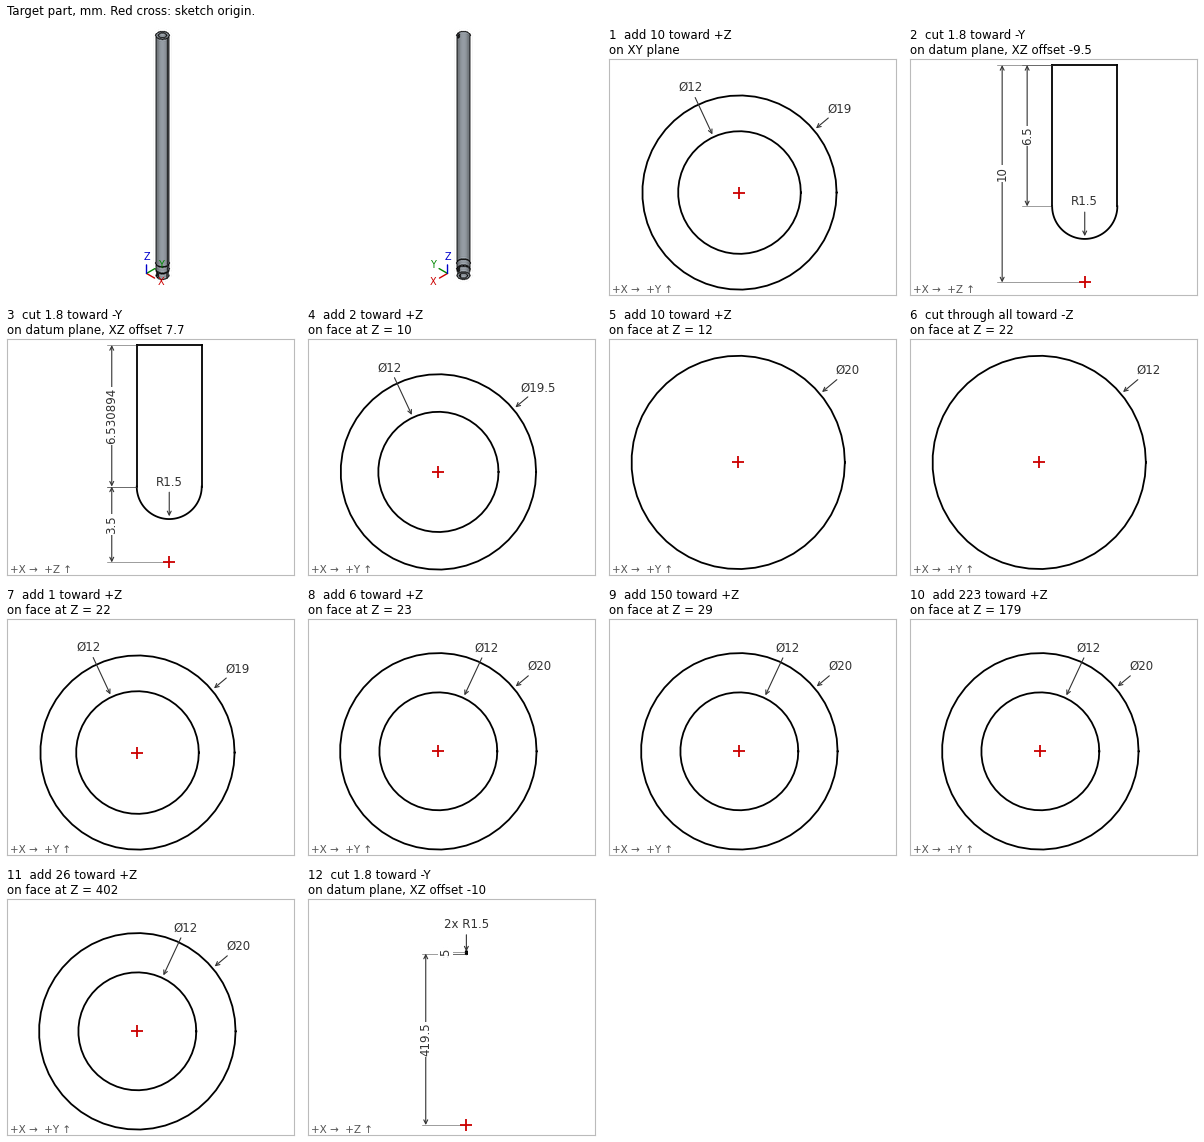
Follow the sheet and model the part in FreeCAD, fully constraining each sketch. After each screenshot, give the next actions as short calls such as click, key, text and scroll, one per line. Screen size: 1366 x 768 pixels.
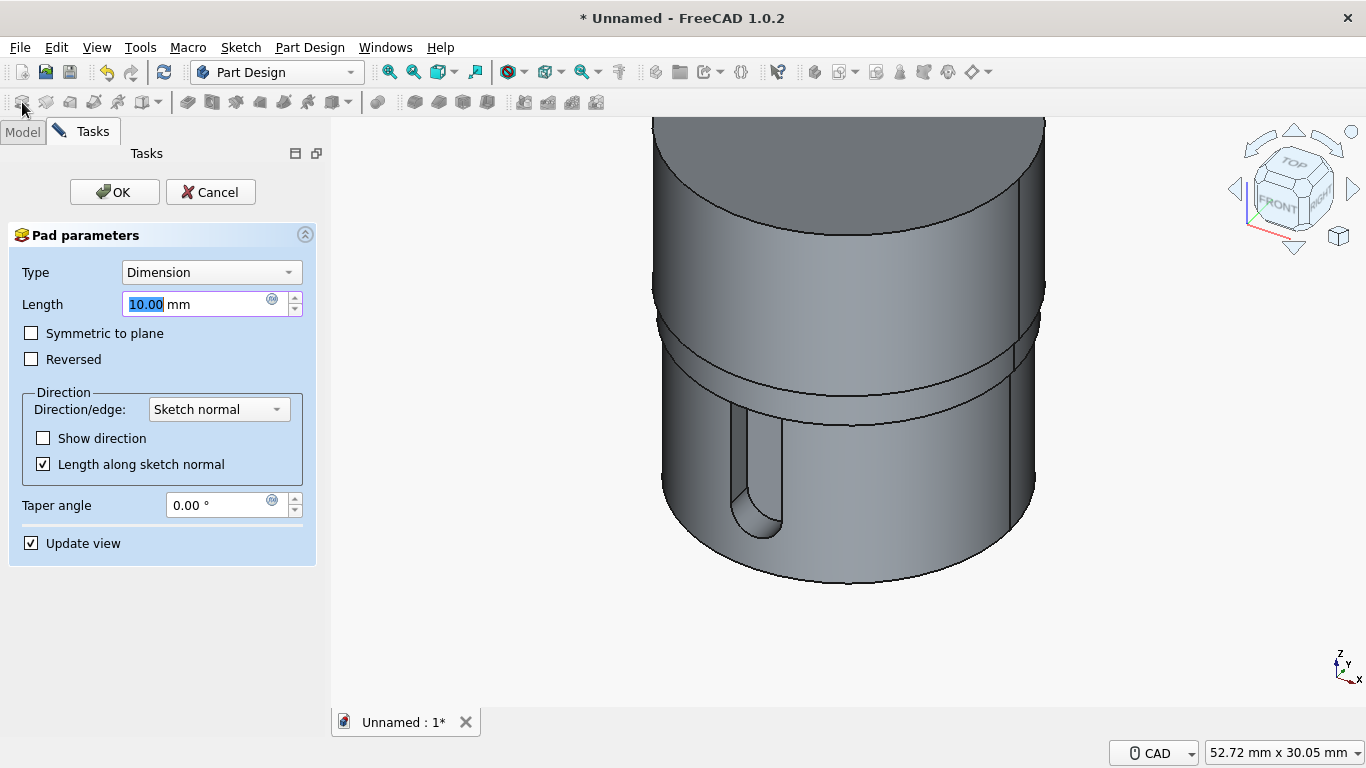
text(10)
key(Tab)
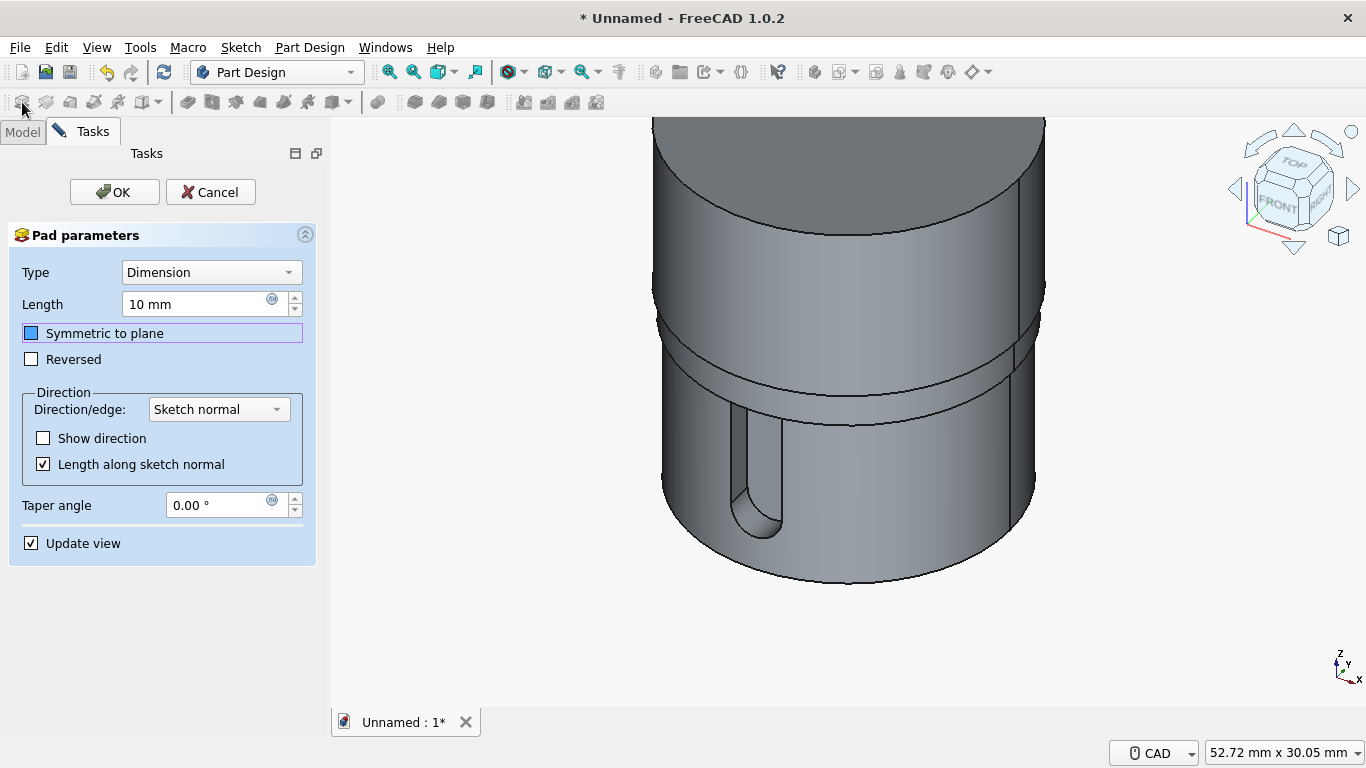
click(115, 192)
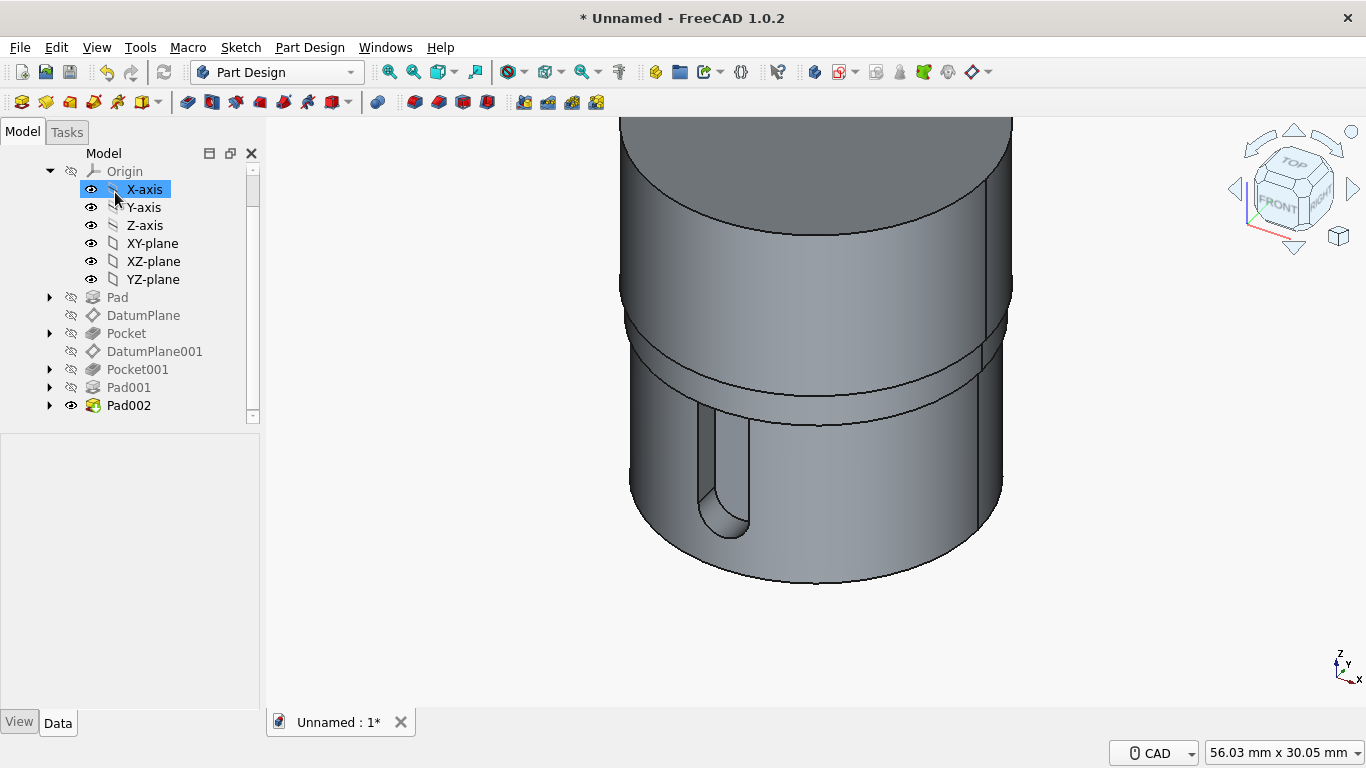
click(390, 72)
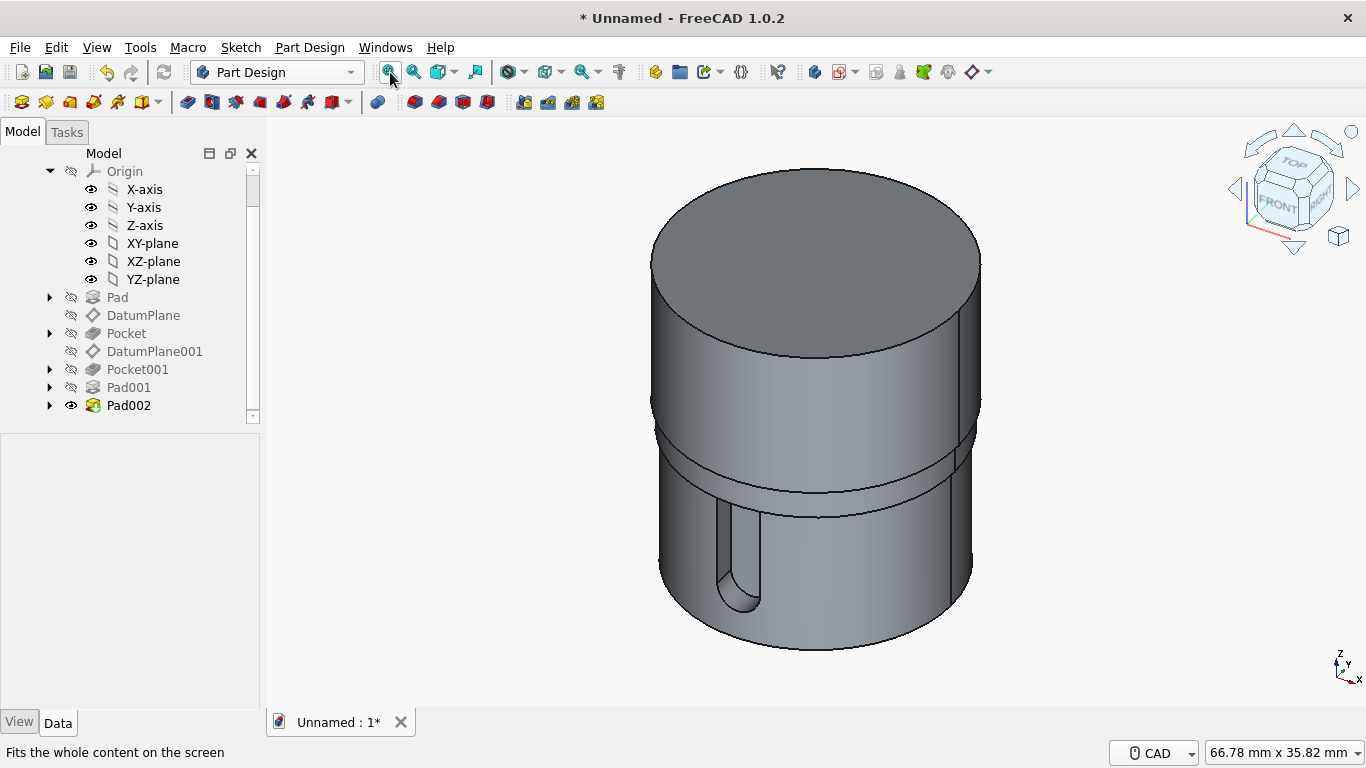
click(816, 263)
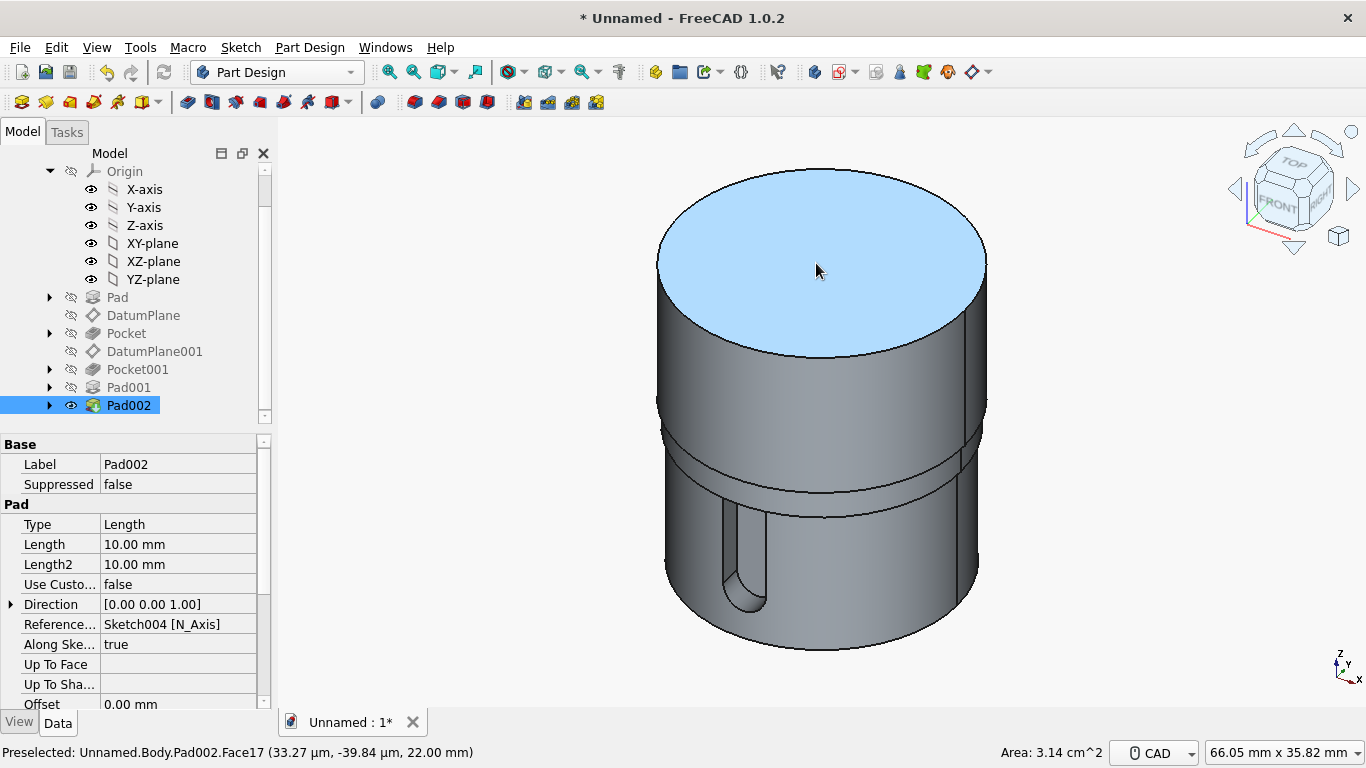
click(840, 72)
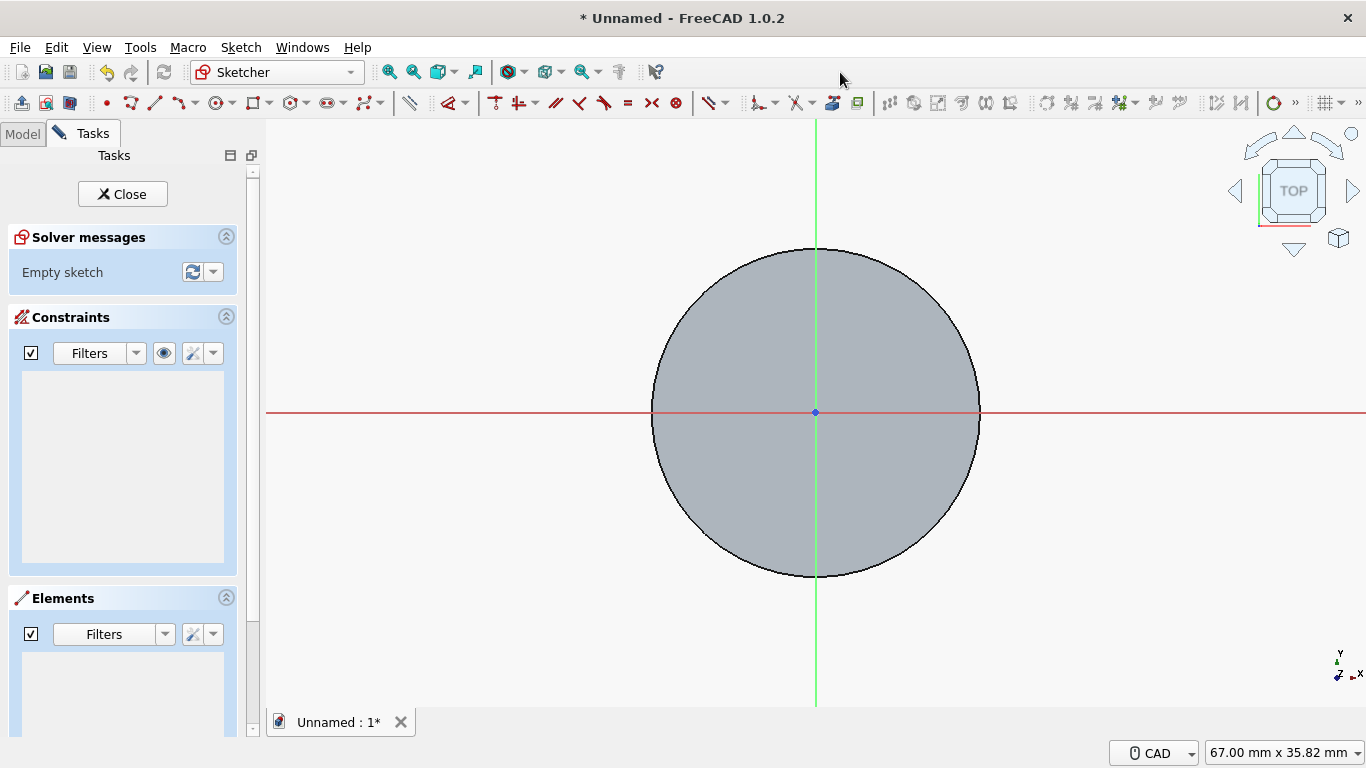
scroll(899, 413, up, 3)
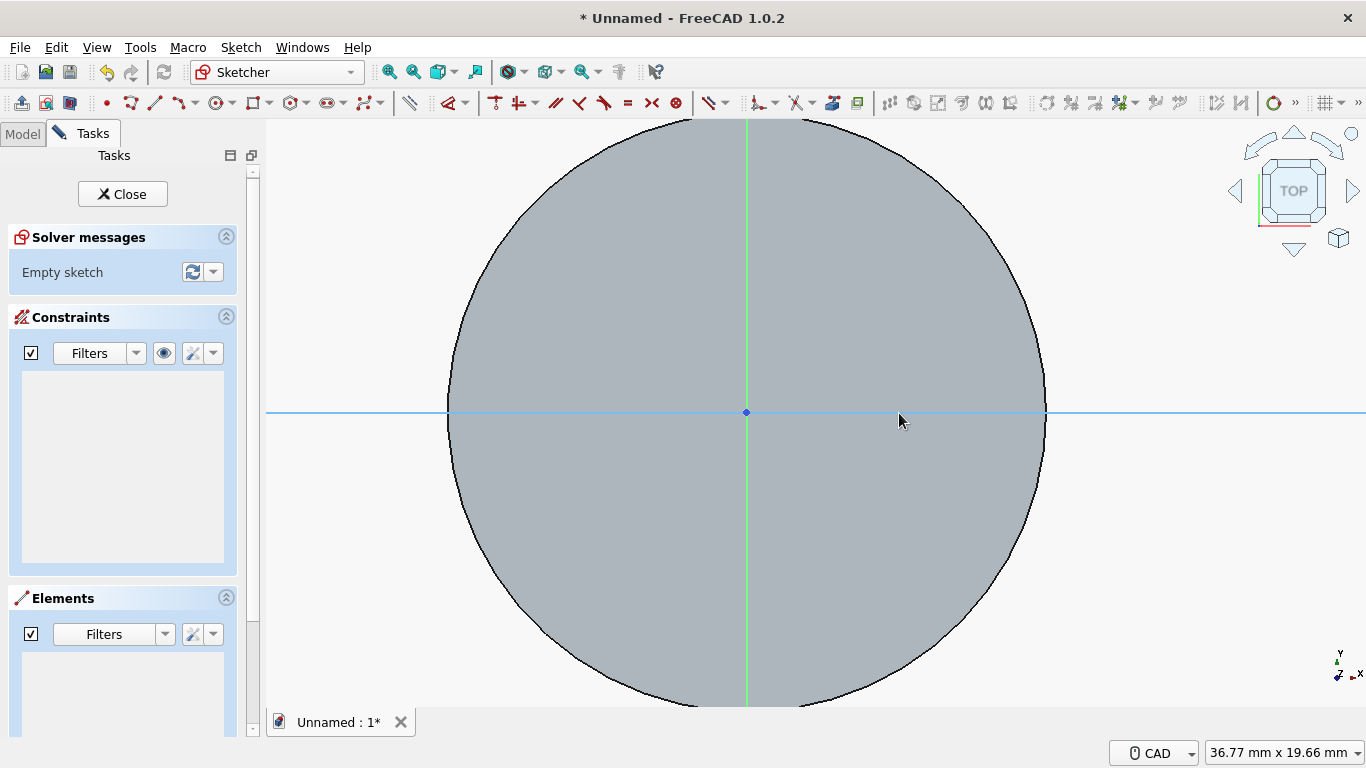
click(216, 104)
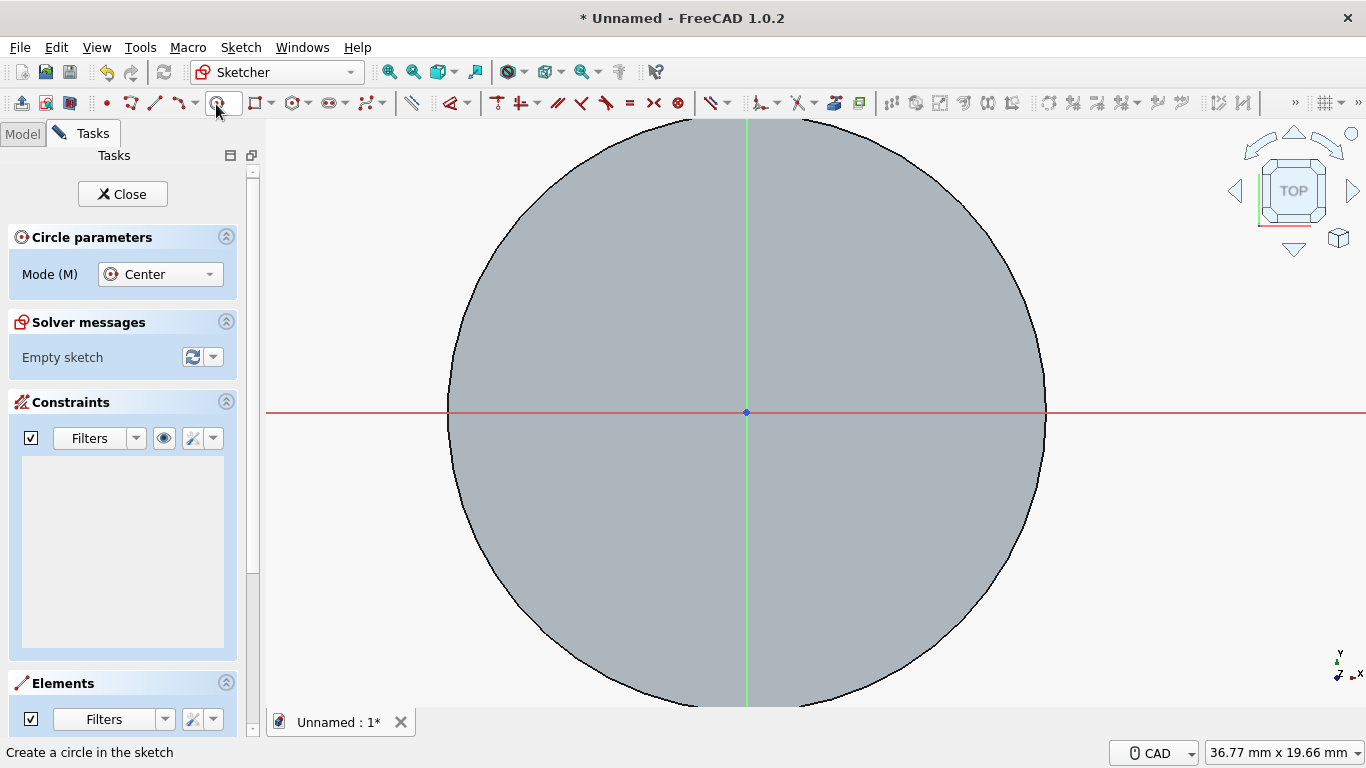
click(747, 413)
click(874, 286)
key(Escape)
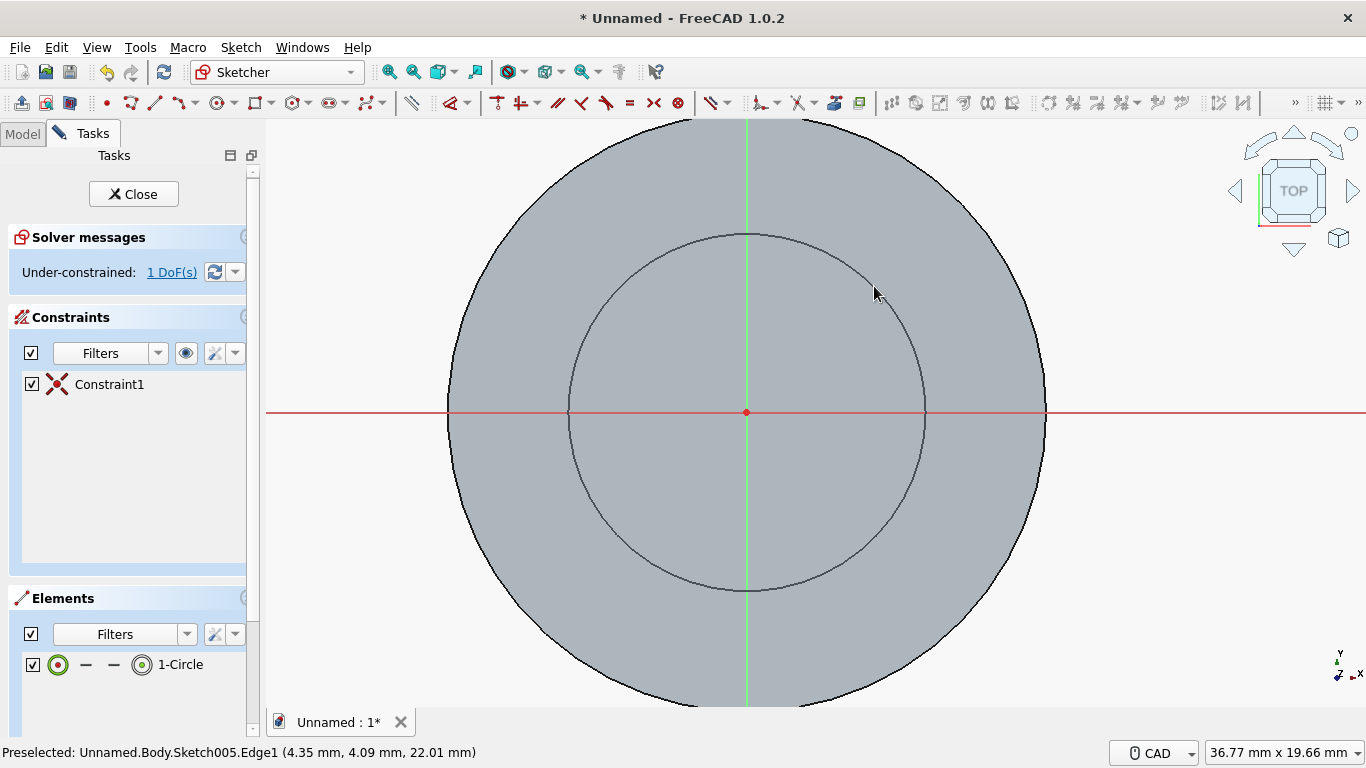
click(450, 104)